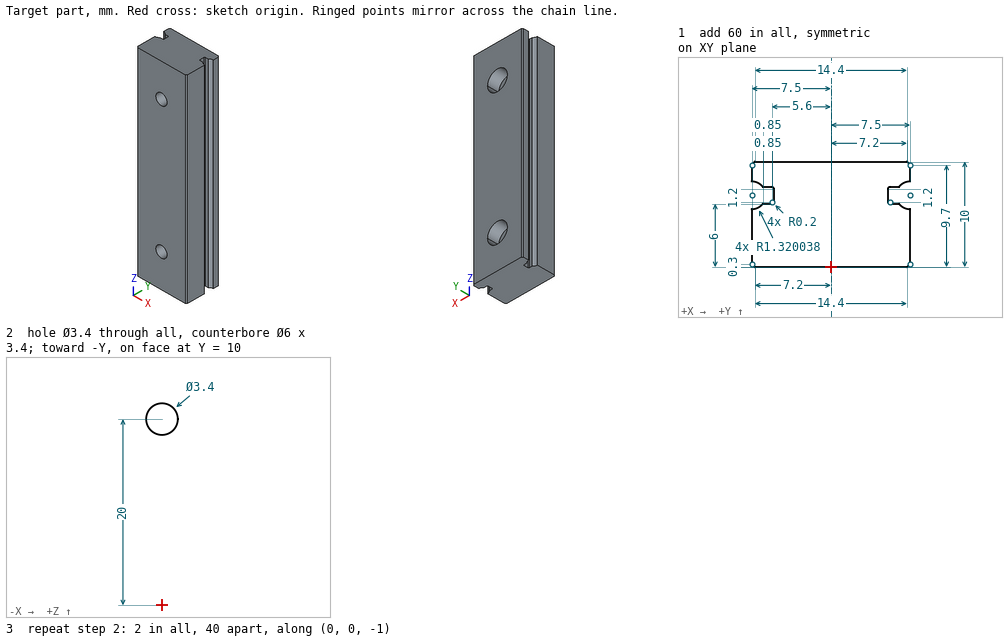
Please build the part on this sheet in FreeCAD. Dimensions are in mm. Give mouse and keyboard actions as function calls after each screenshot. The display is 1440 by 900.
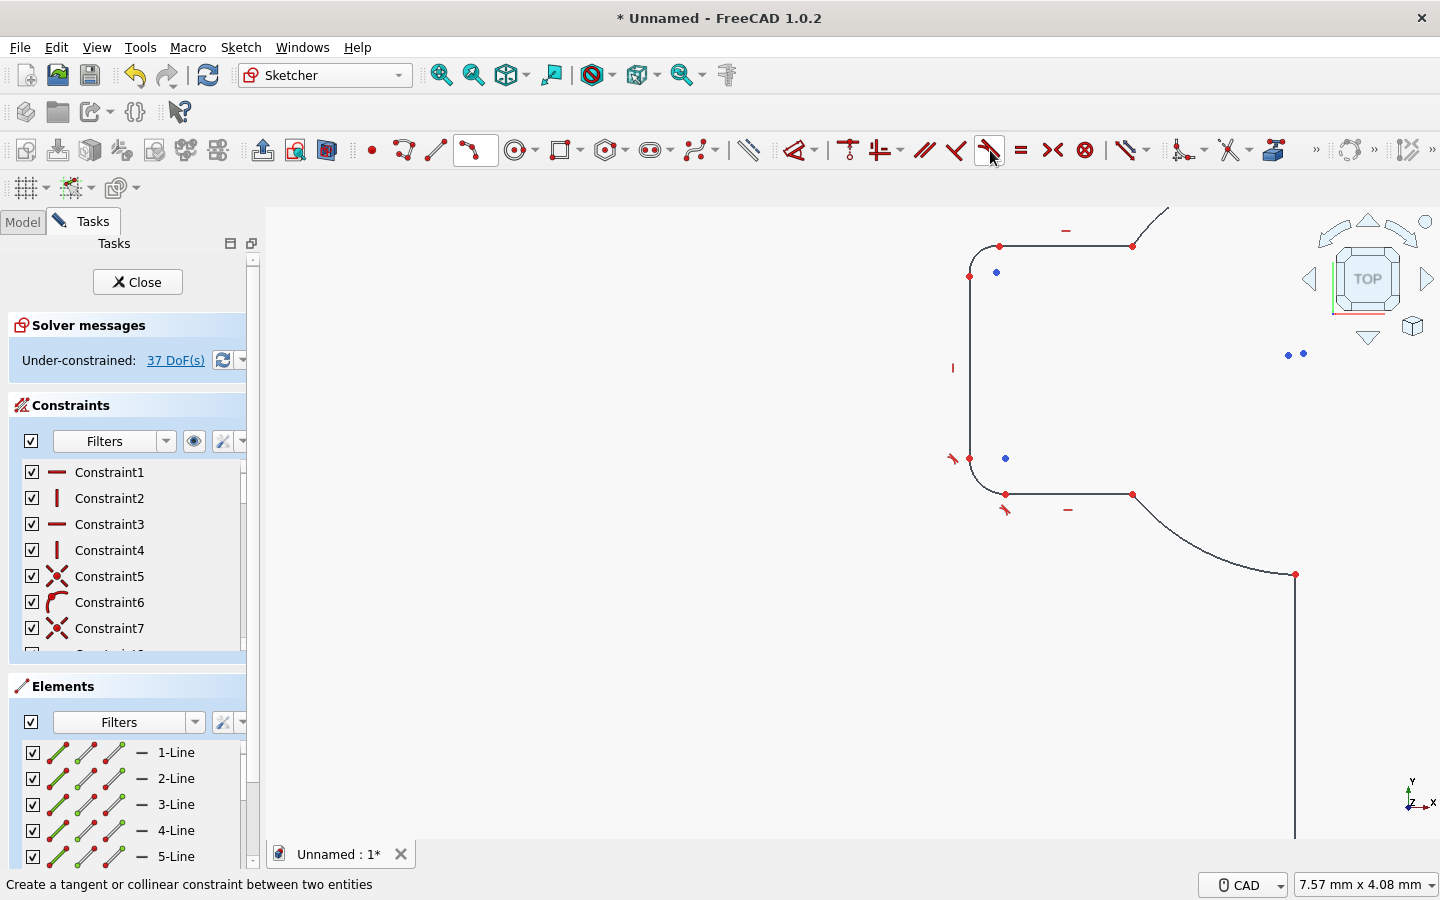
scroll(998, 483, down, 7)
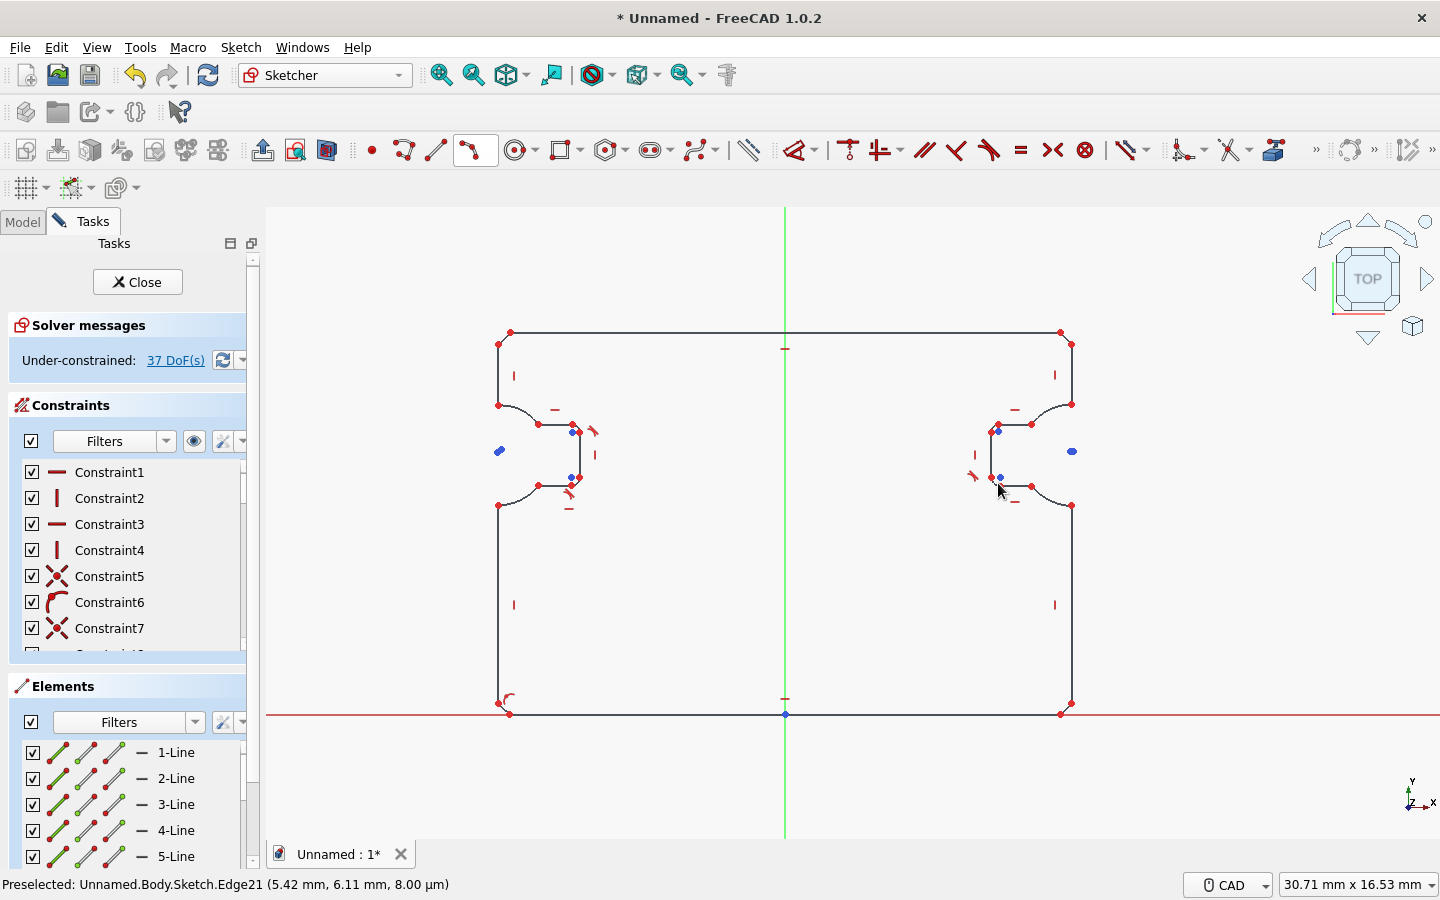
click(992, 464)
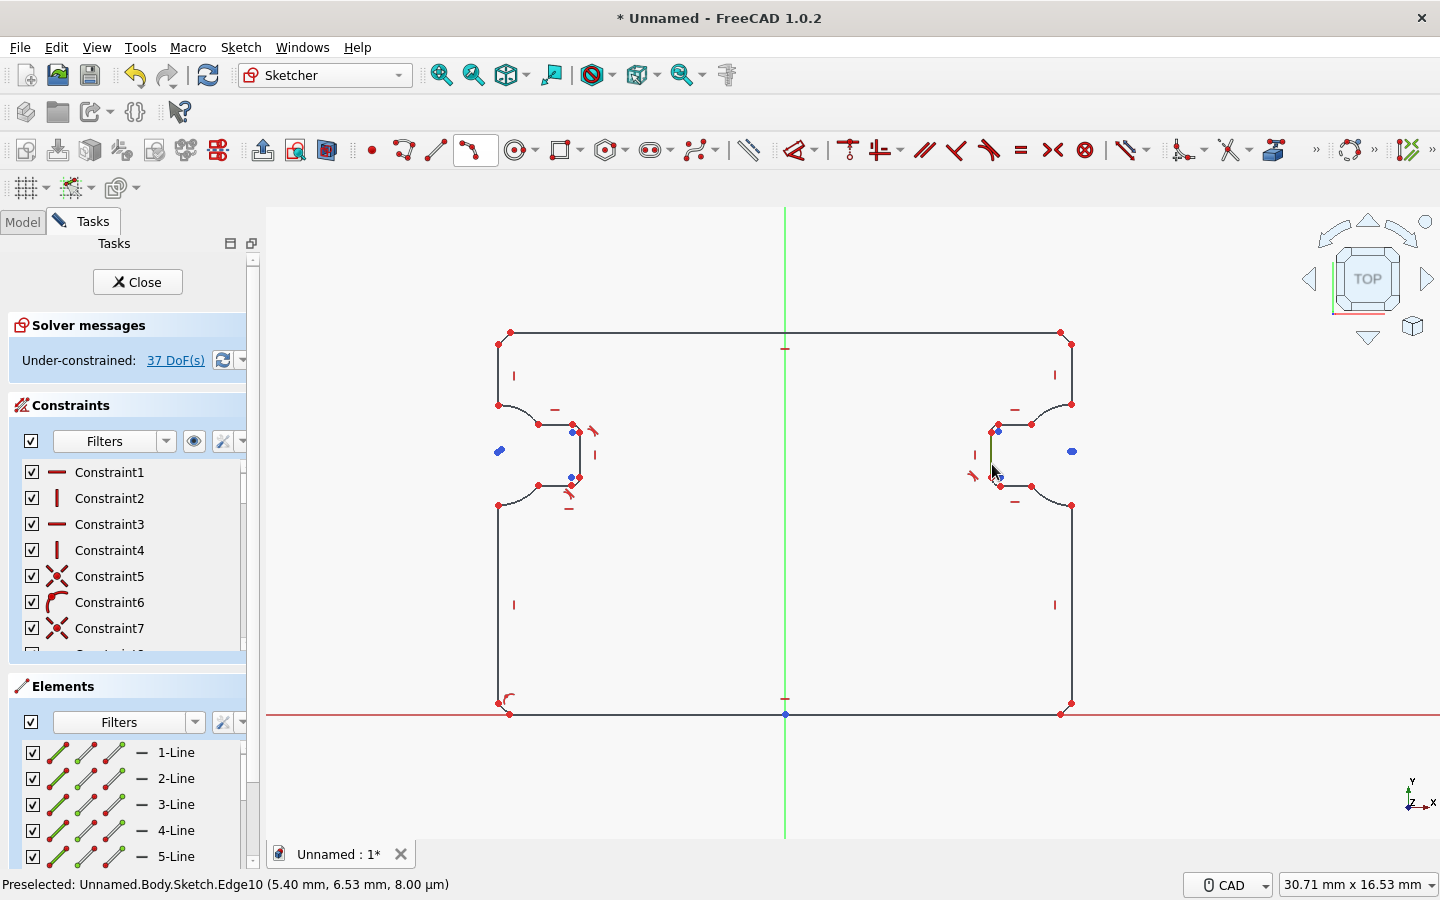
scroll(993, 427, up, 5)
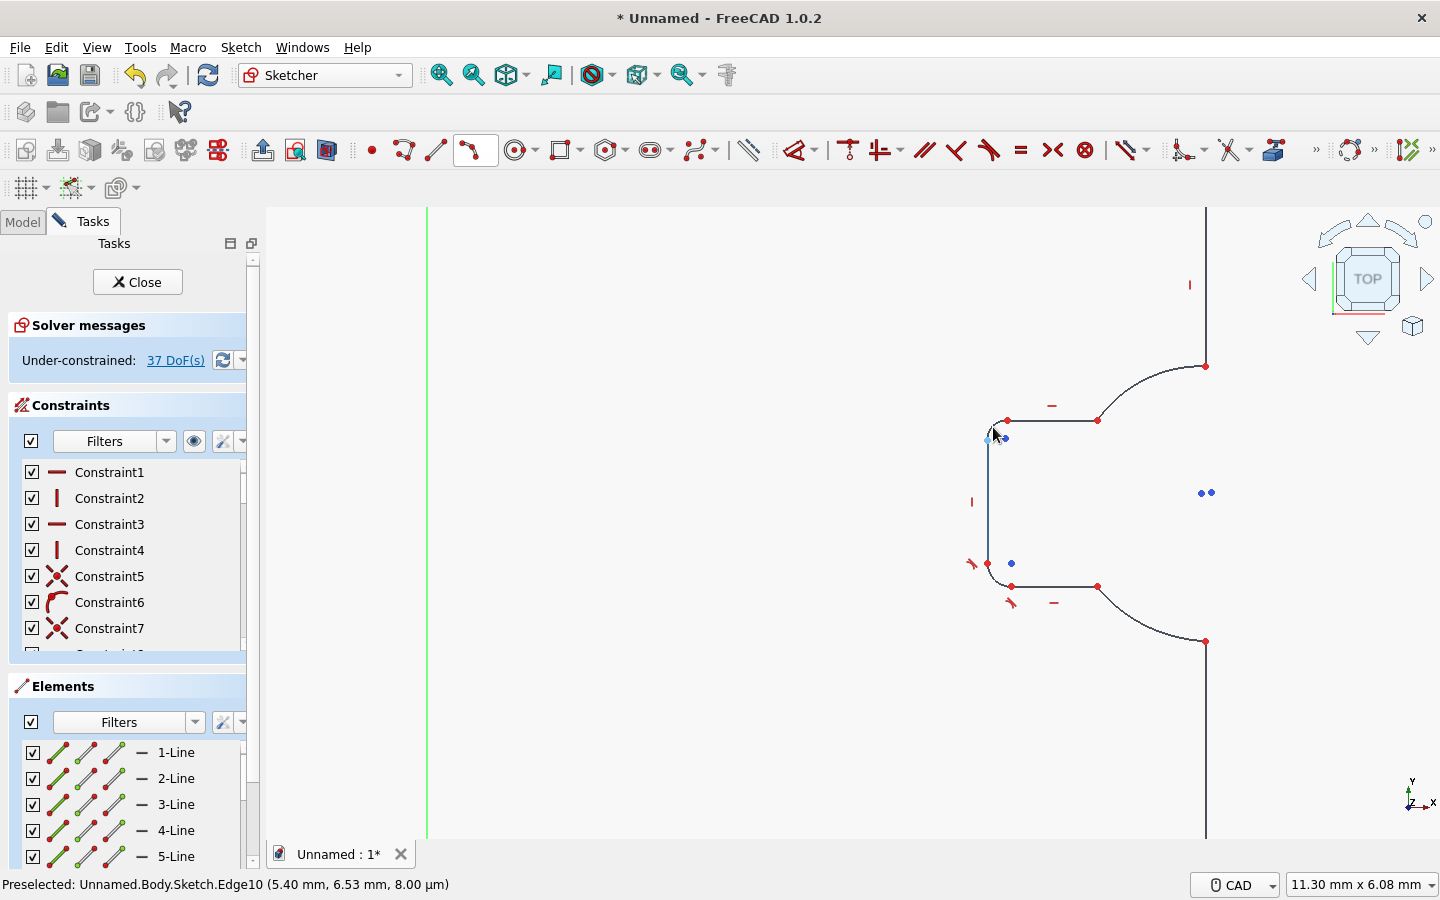
click(993, 426)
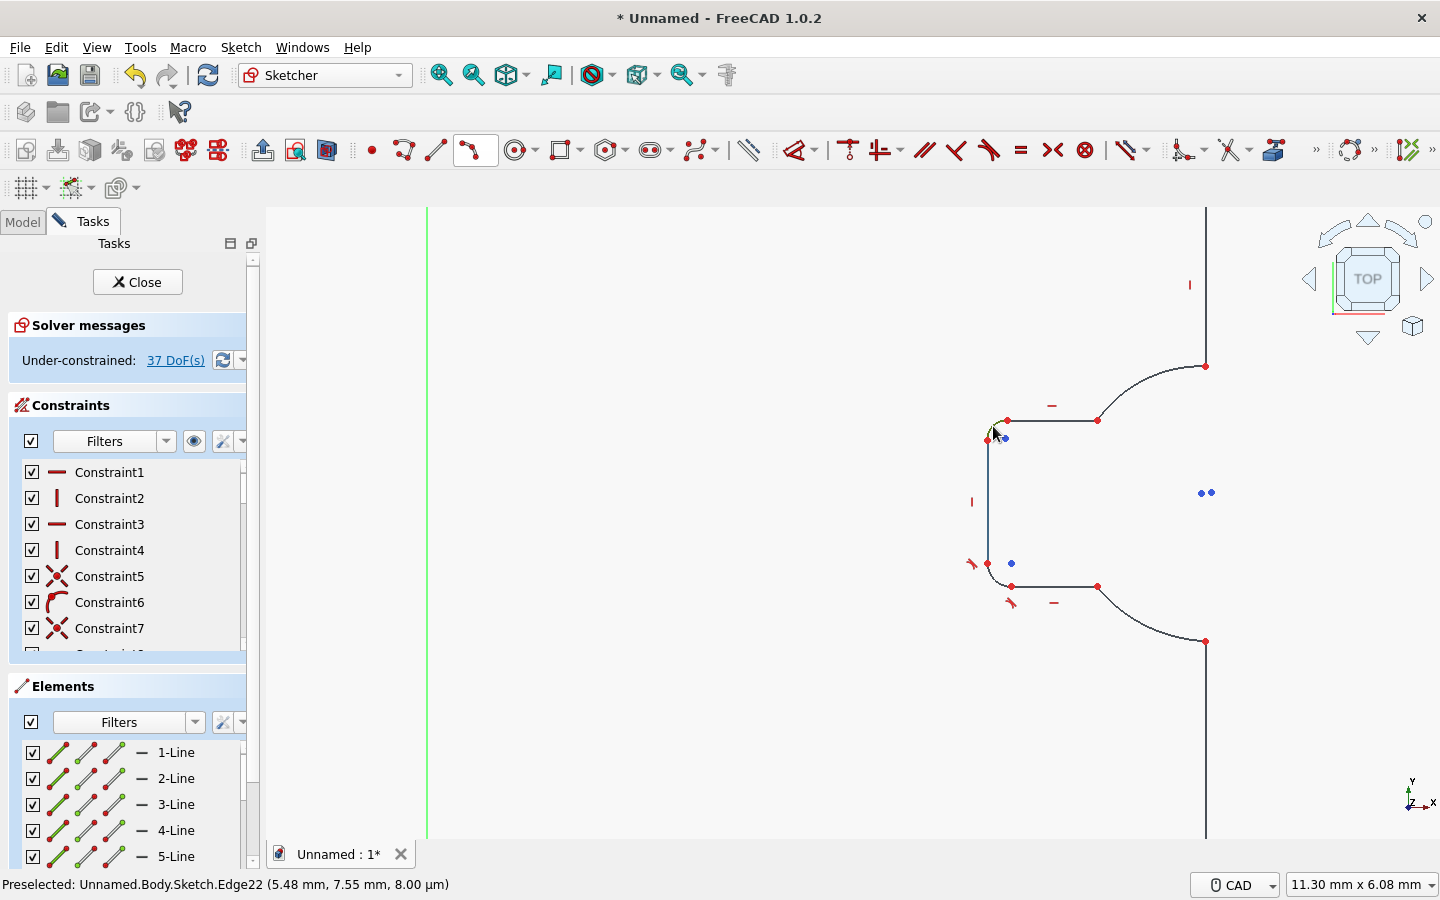
click(990, 150)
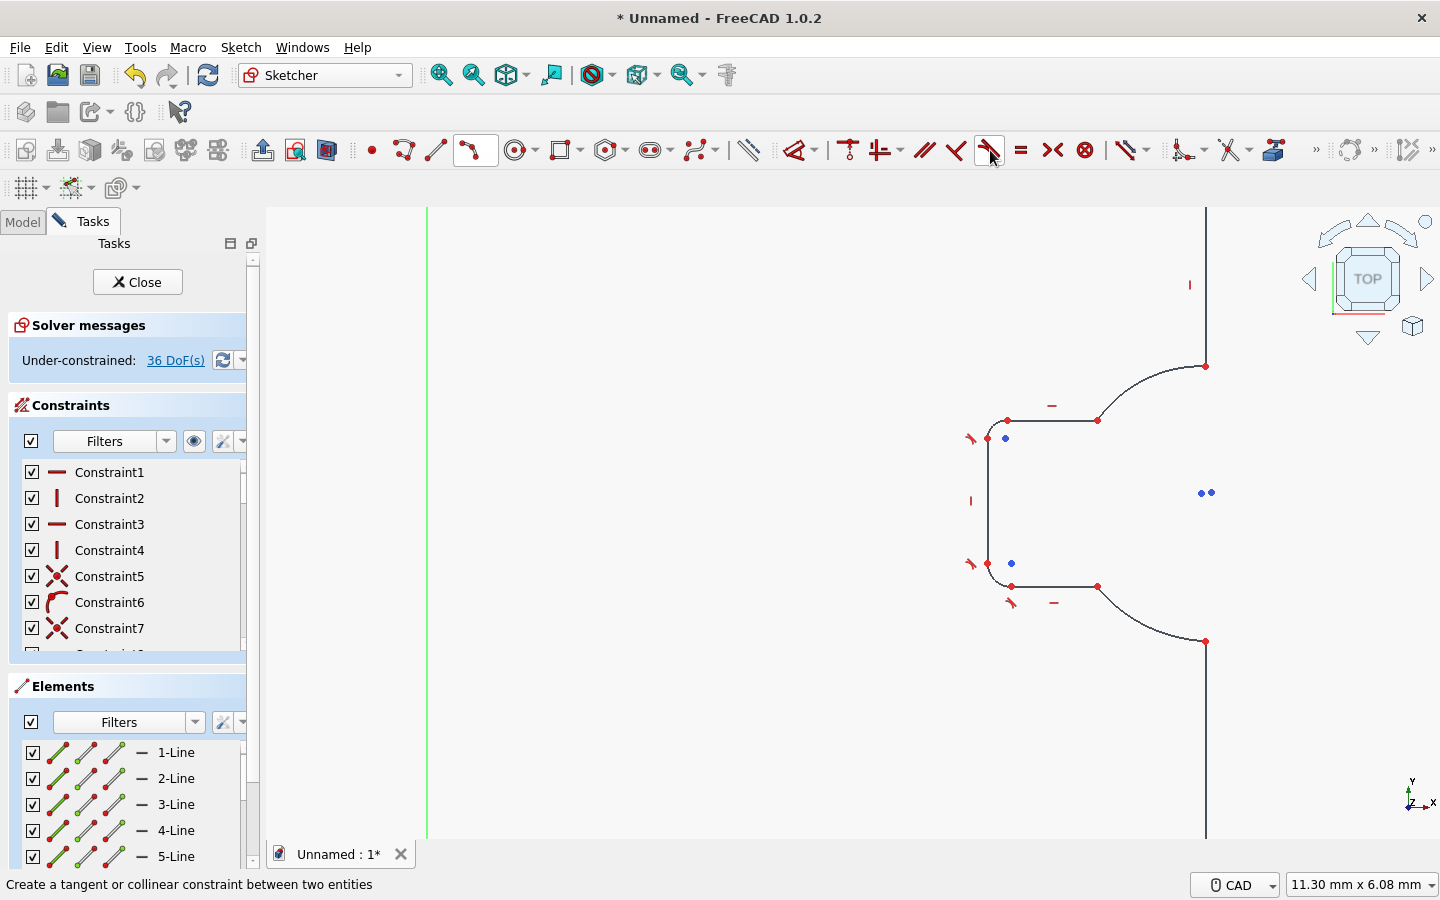
click(1035, 421)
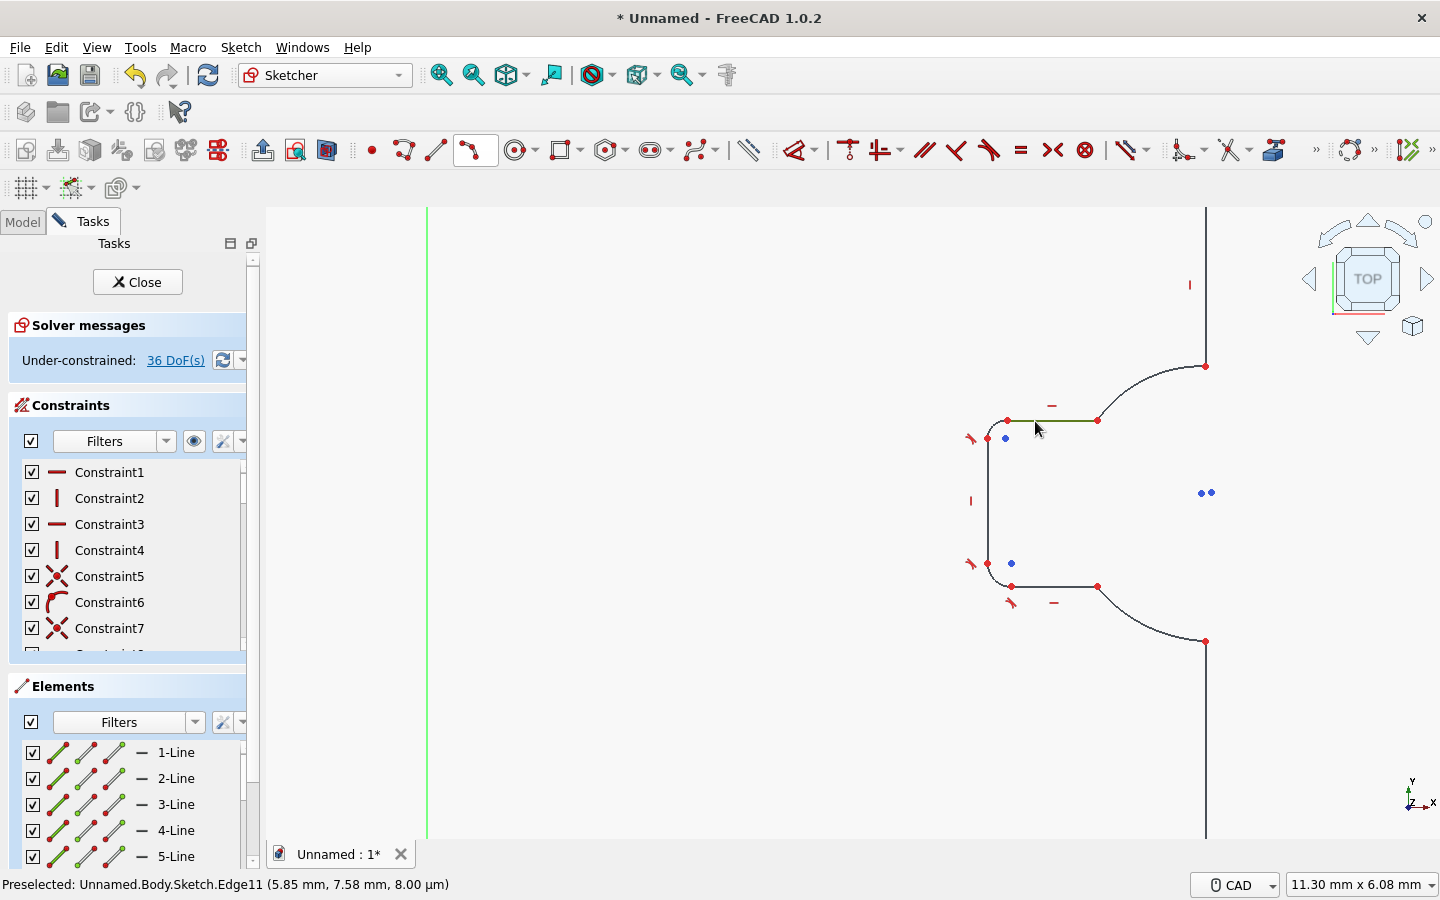
scroll(999, 422, up, 3)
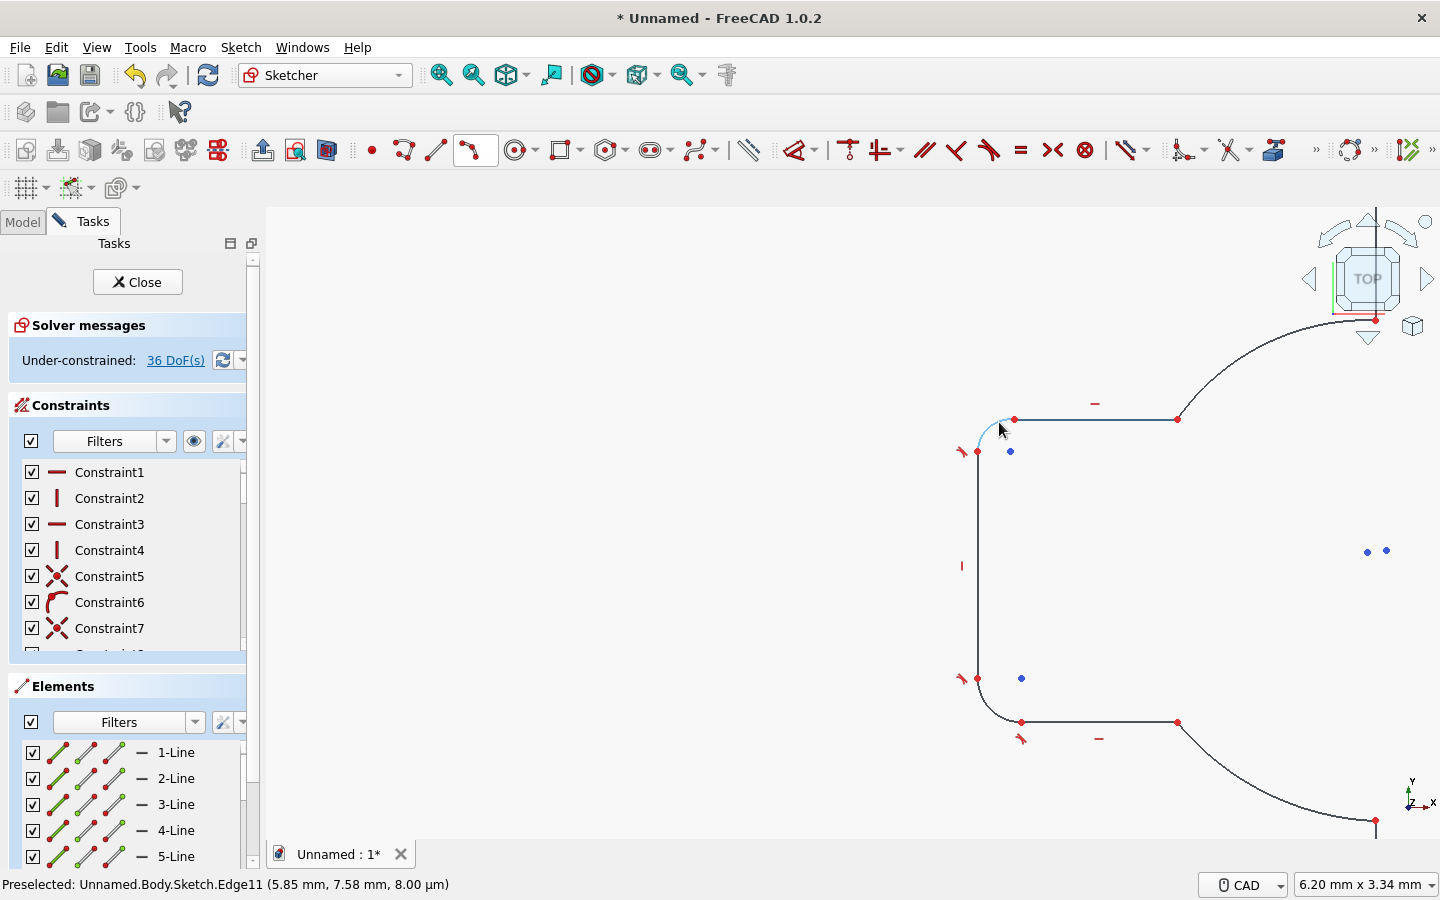
click(998, 422)